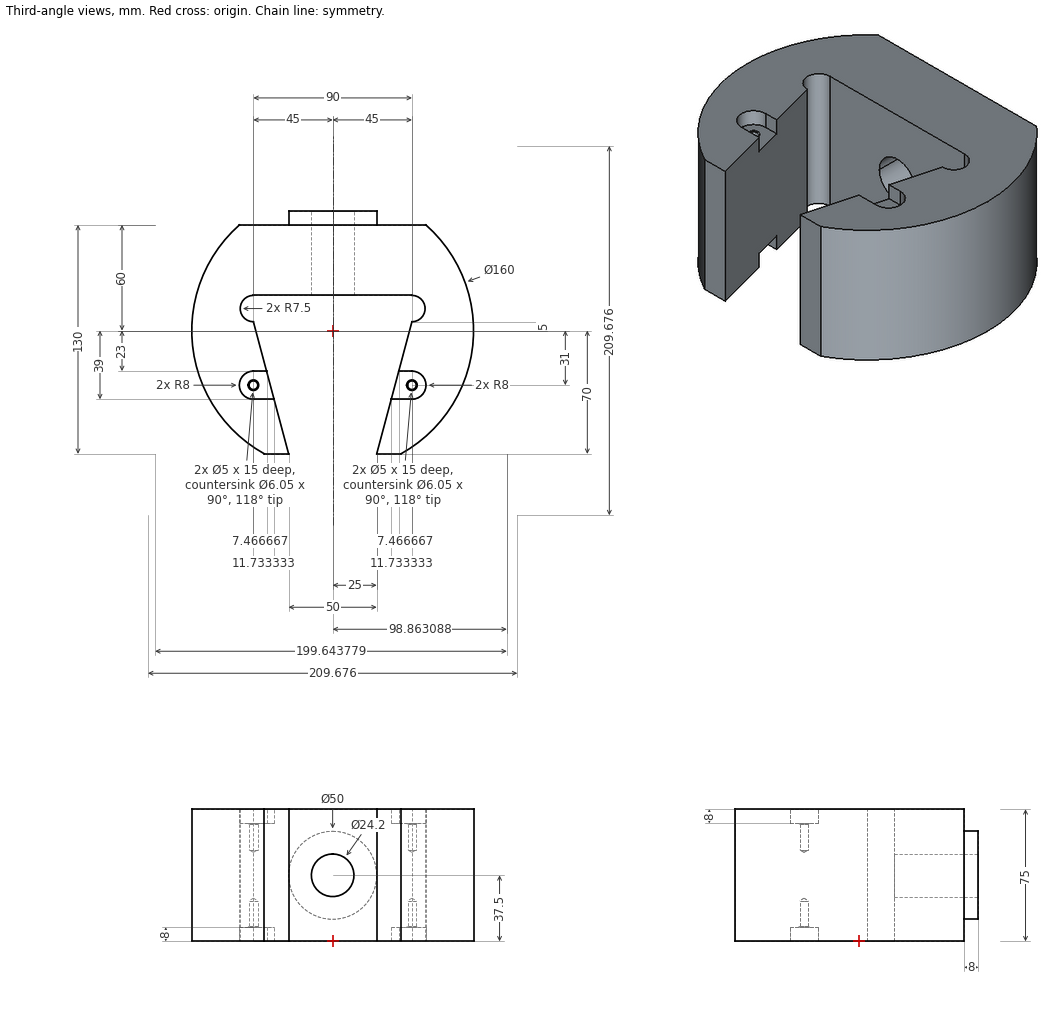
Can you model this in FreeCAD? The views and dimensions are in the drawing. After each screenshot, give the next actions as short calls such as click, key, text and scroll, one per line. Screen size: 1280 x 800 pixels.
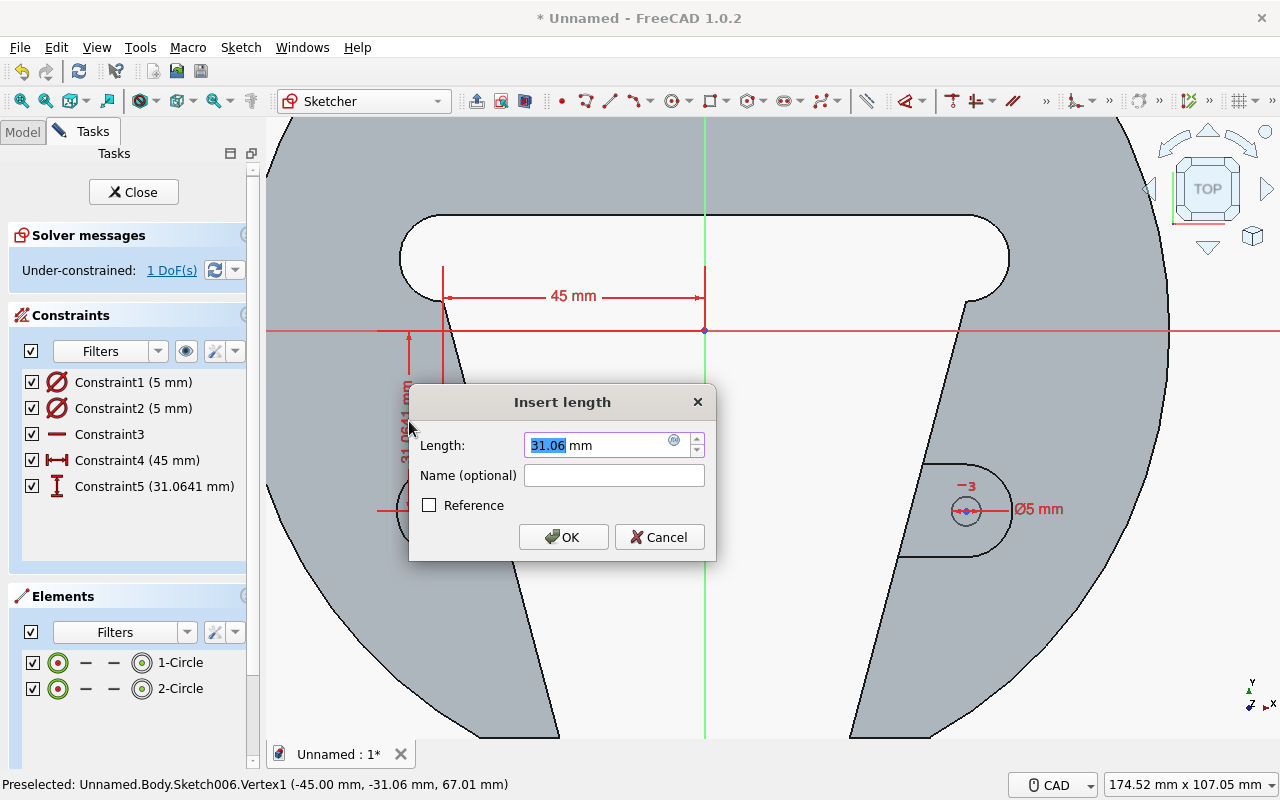
text(31)
key(Return)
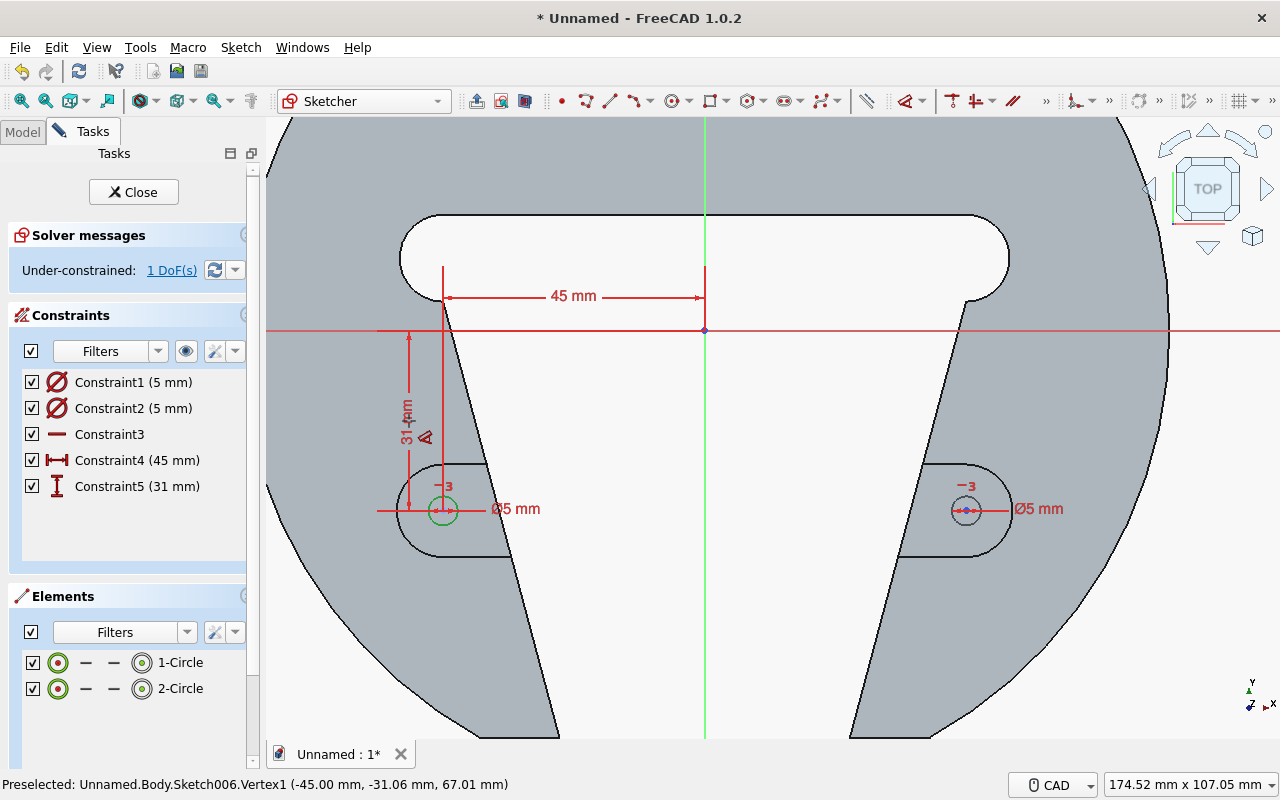
click(966, 511)
click(835, 297)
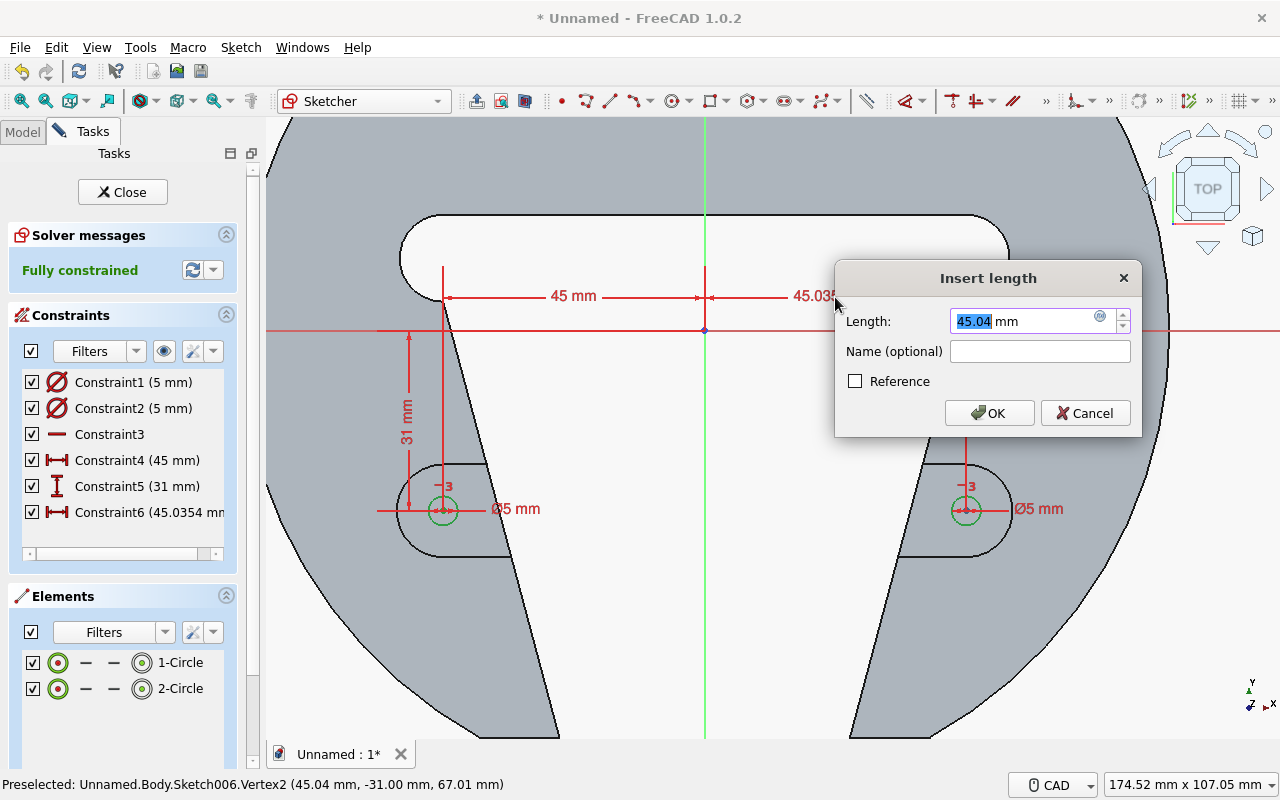
text(45)
key(Return)
key(Escape)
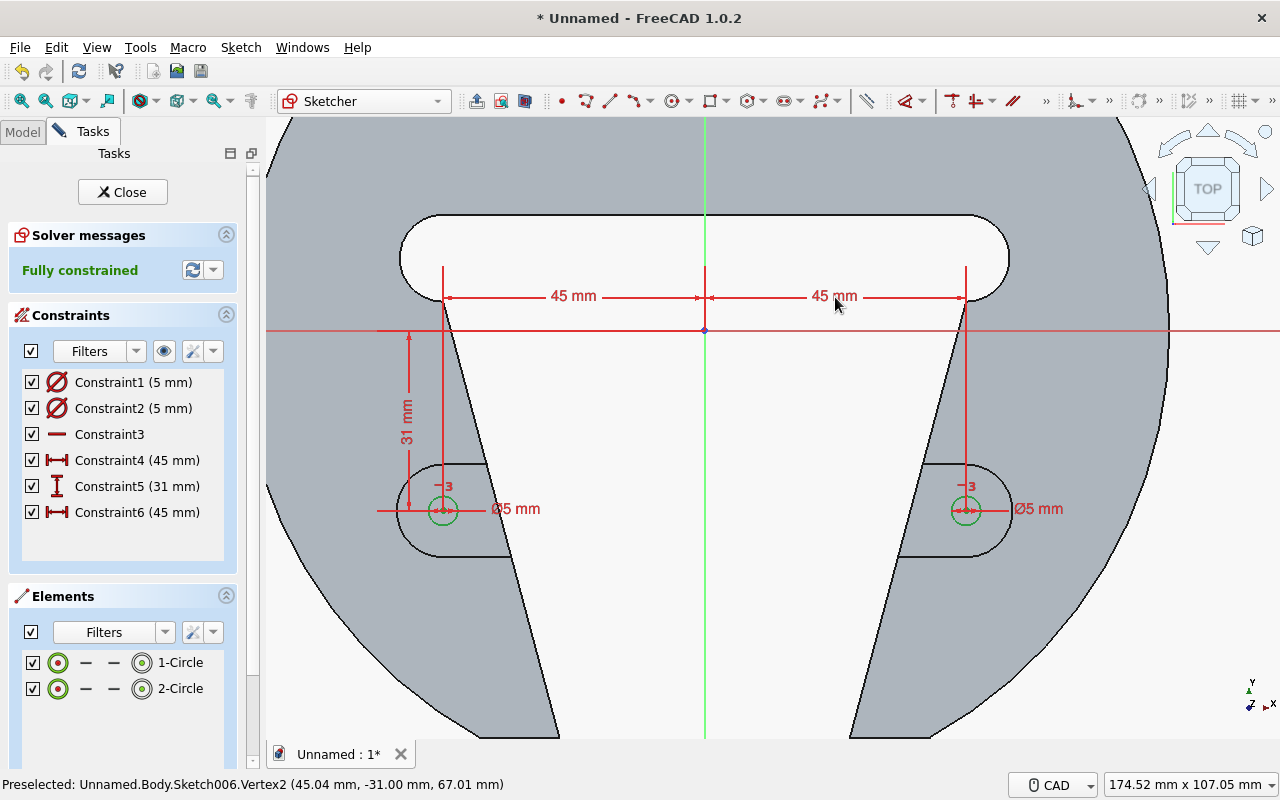
click(123, 192)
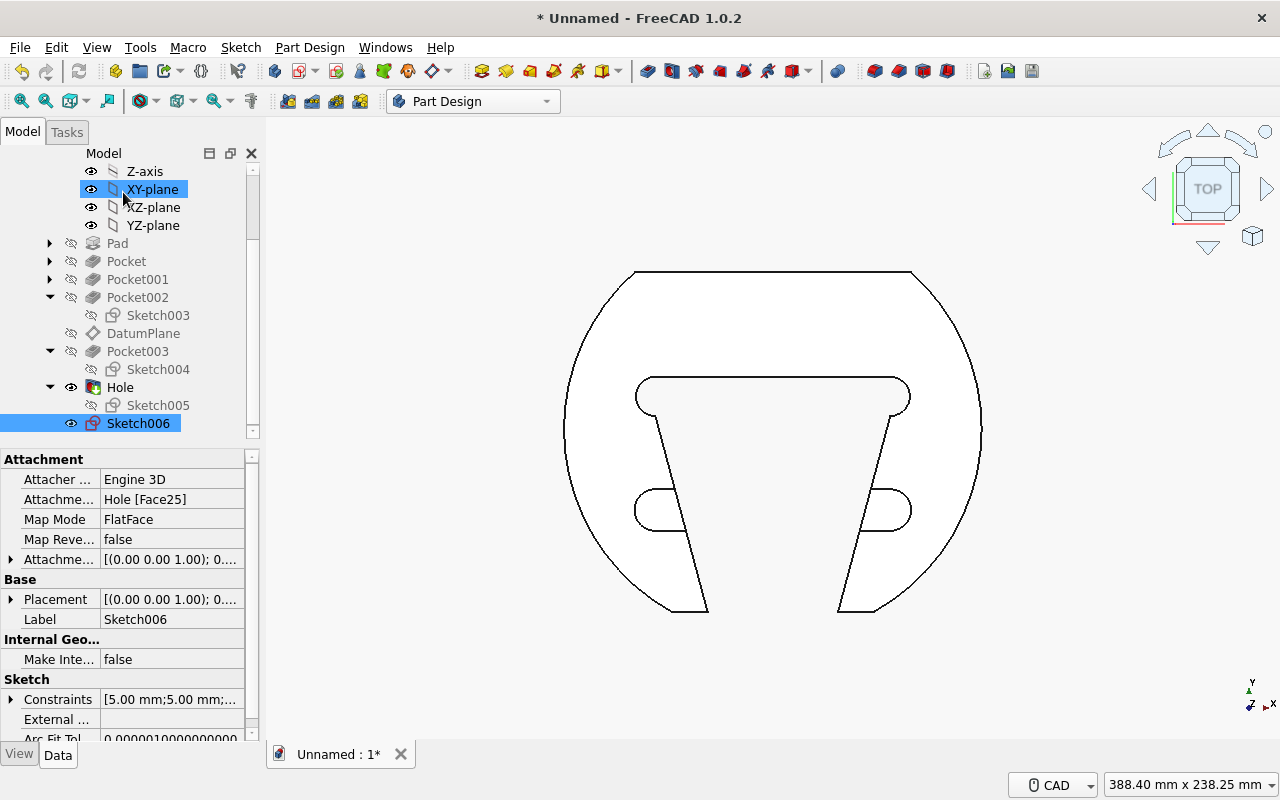
click(672, 72)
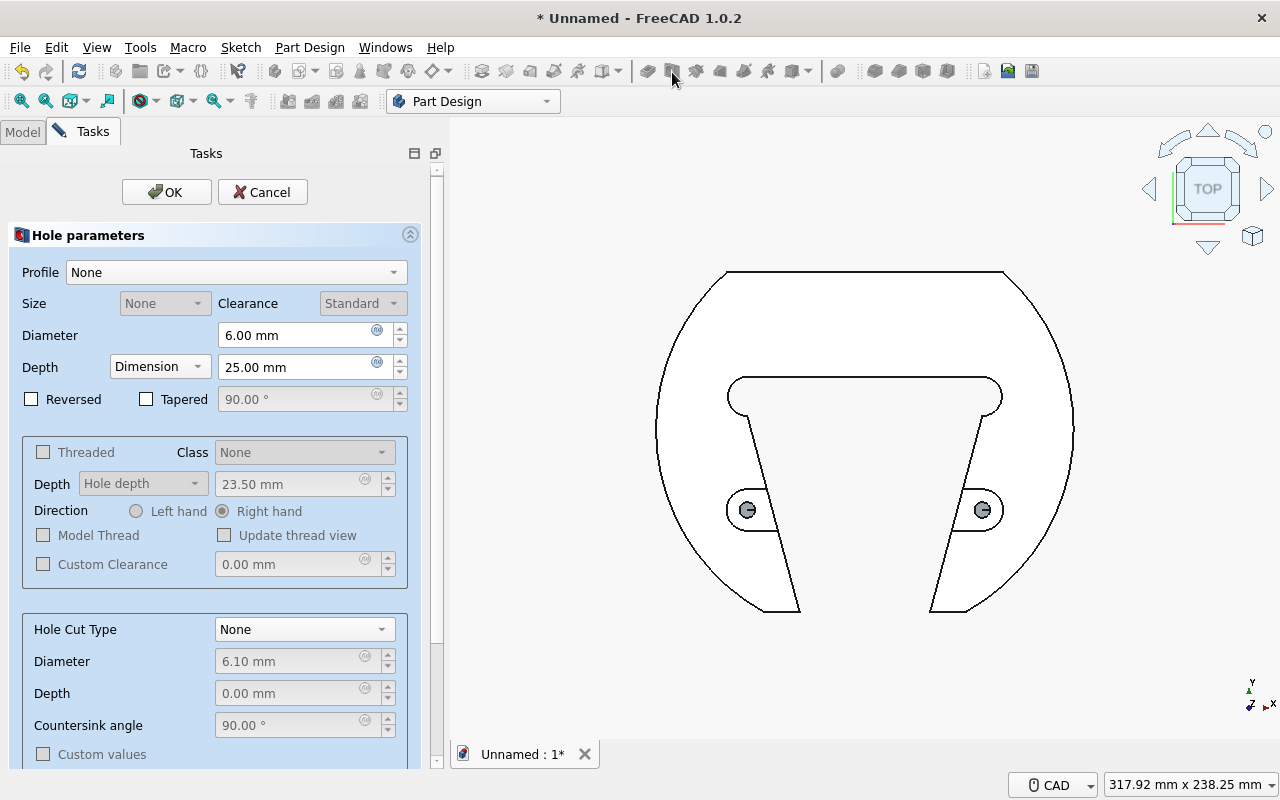
triple_click(305, 335)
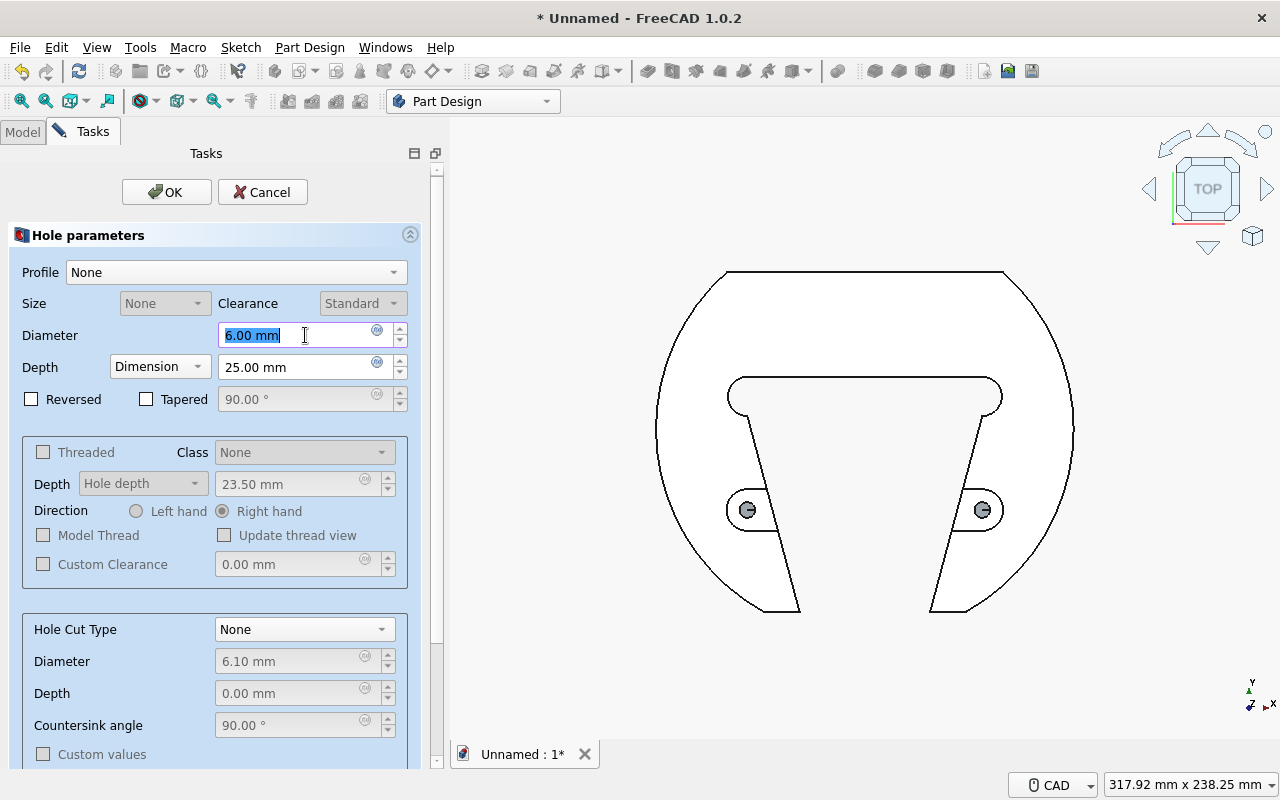
text(5)
key(Tab)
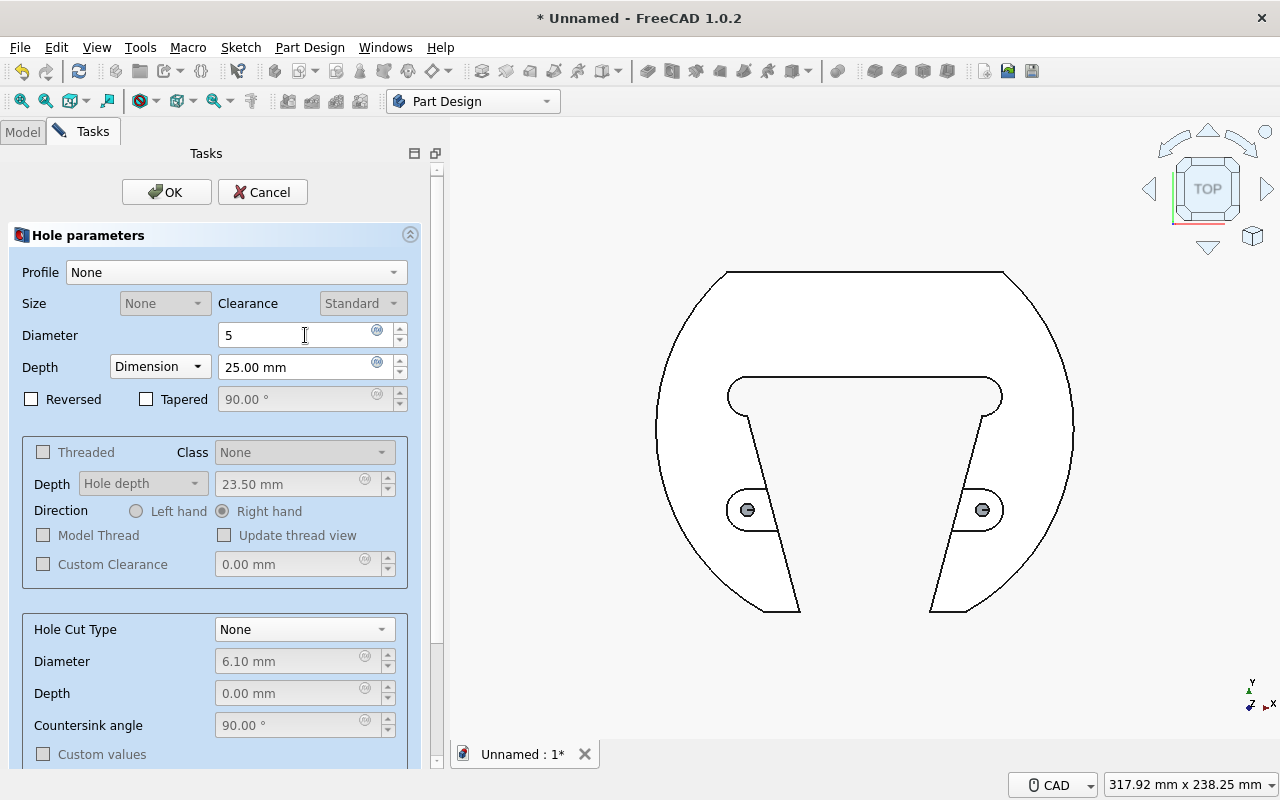
triple_click(305, 367)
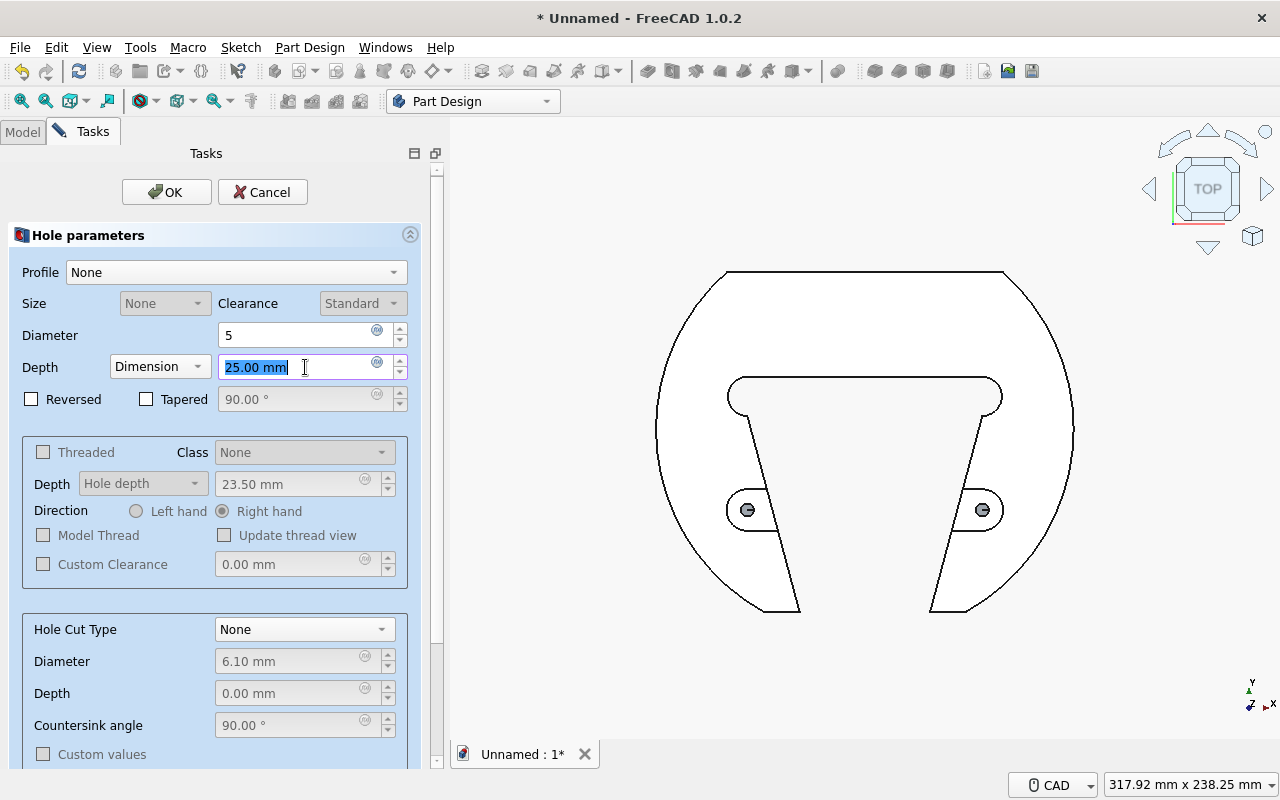
text(15)
key(Tab)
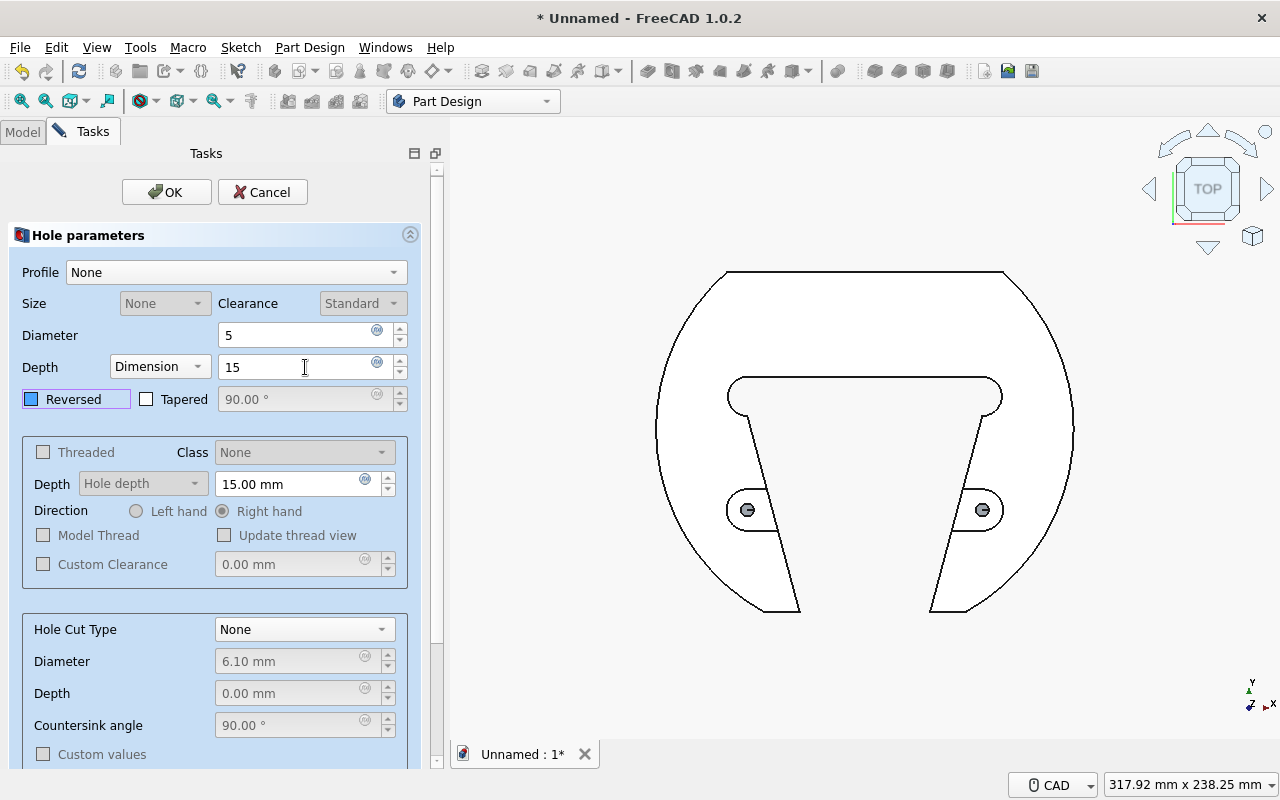
click(306, 630)